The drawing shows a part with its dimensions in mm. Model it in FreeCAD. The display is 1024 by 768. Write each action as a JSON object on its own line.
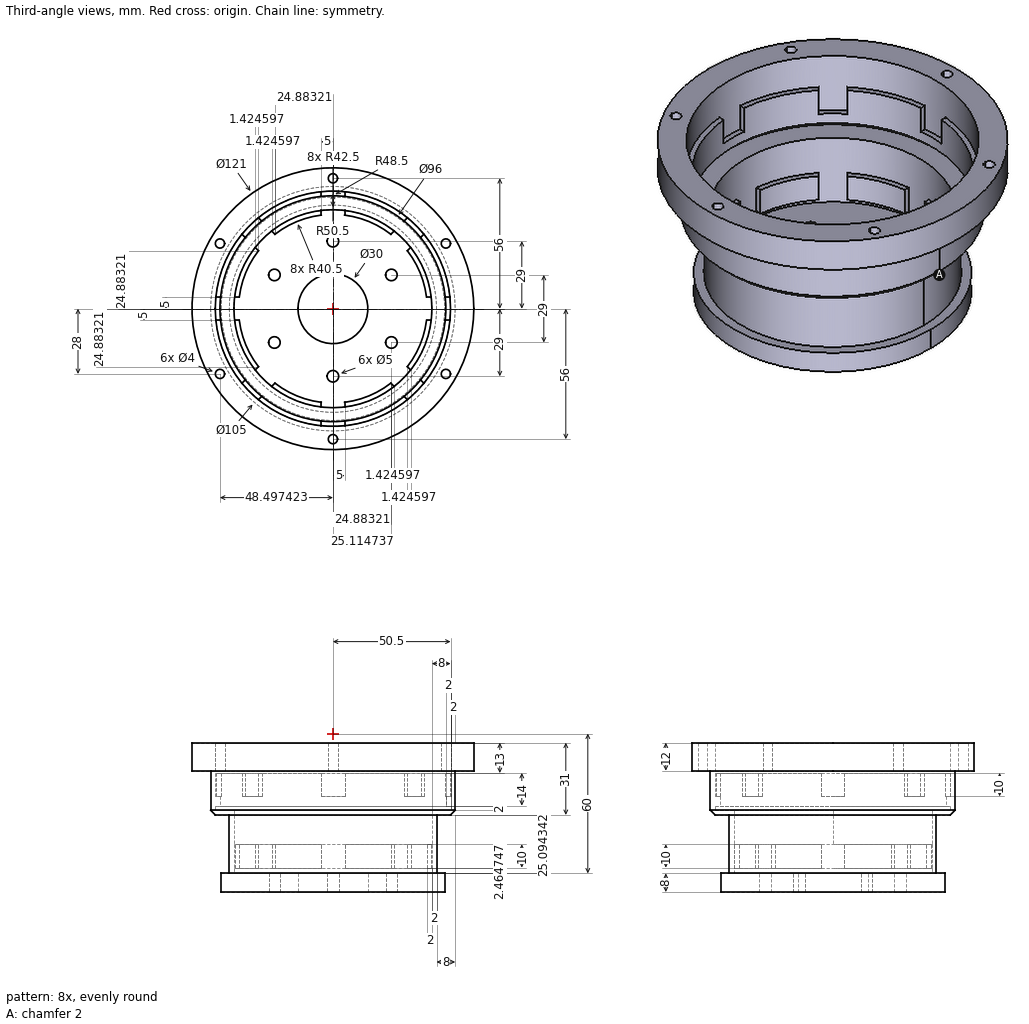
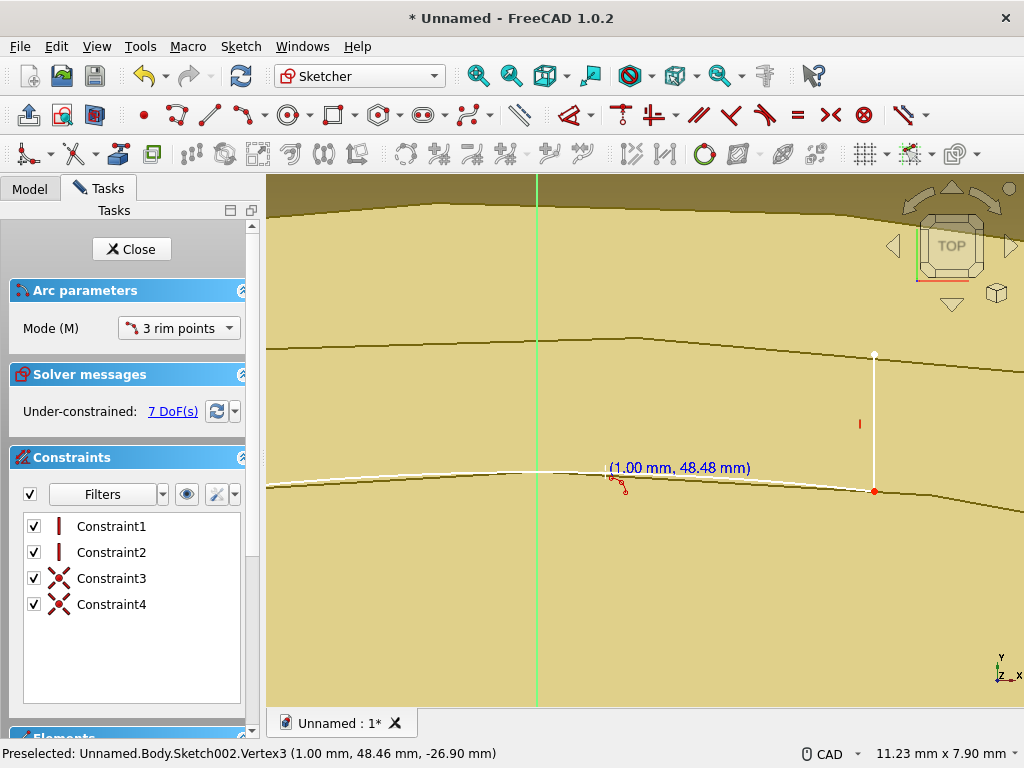
{"action": "scroll", "coordinate": [624, 474], "scroll_direction": "down", "scroll_amount": 3}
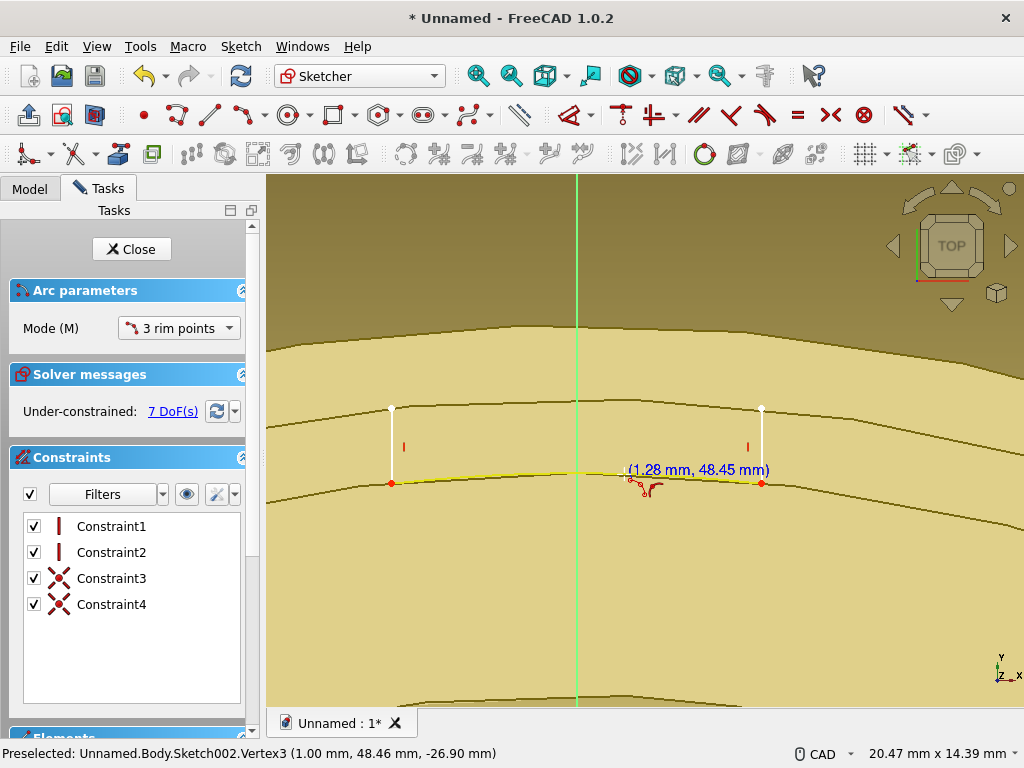
{"action": "left_click", "coordinate": [762, 409]}
{"action": "left_click", "coordinate": [392, 409]}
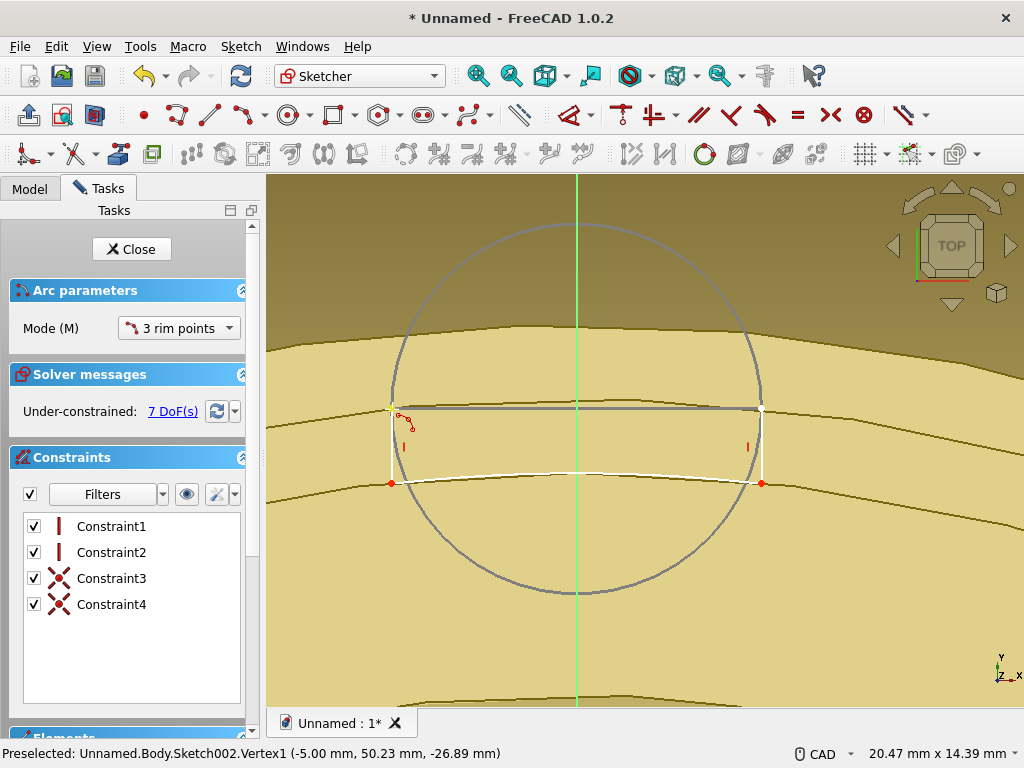
{"action": "scroll", "coordinate": [614, 399], "scroll_direction": "up", "scroll_amount": 3}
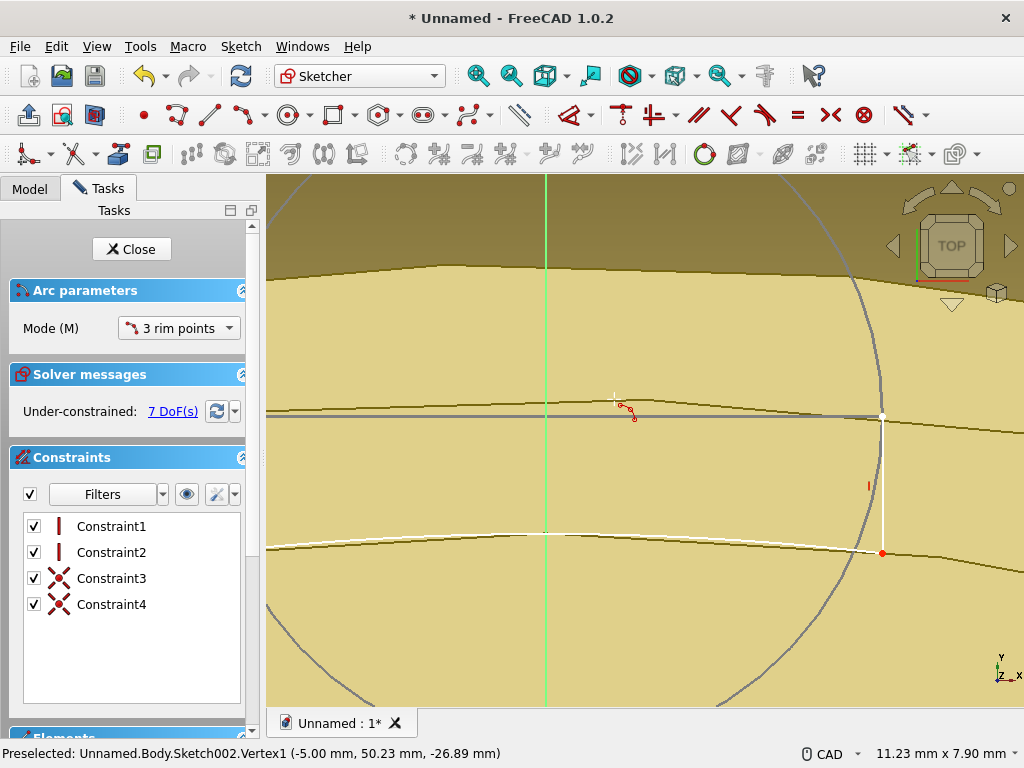
{"action": "left_click", "coordinate": [613, 399]}
{"action": "key", "text": "Escape"}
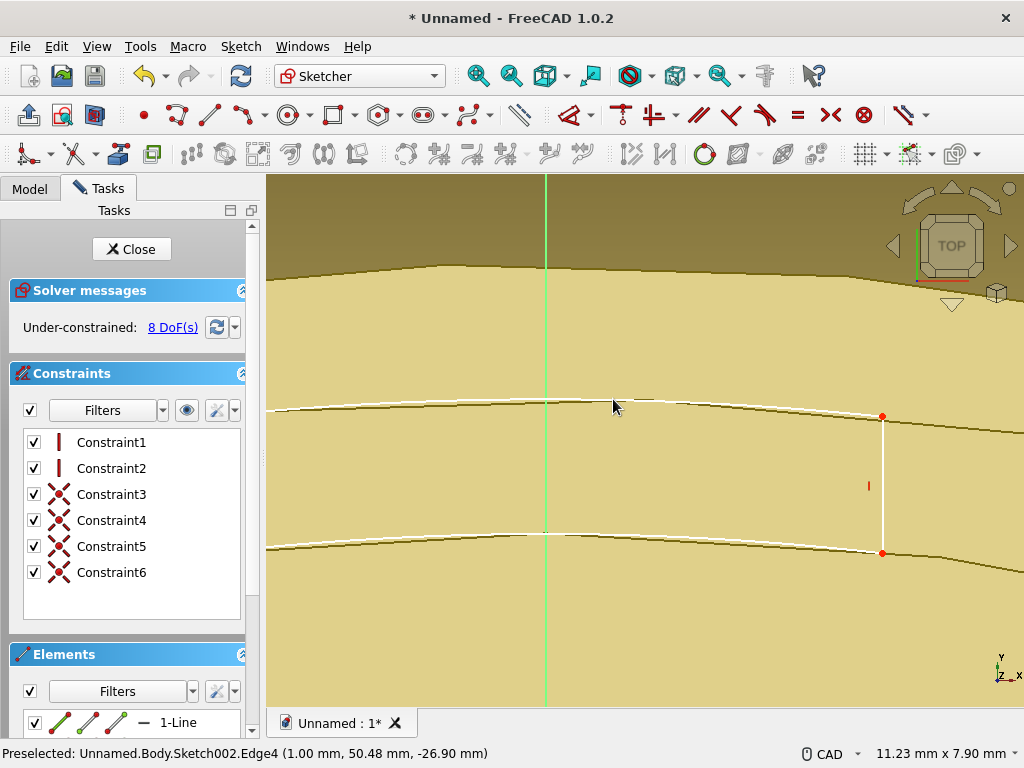
{"action": "left_click", "coordinate": [681, 537]}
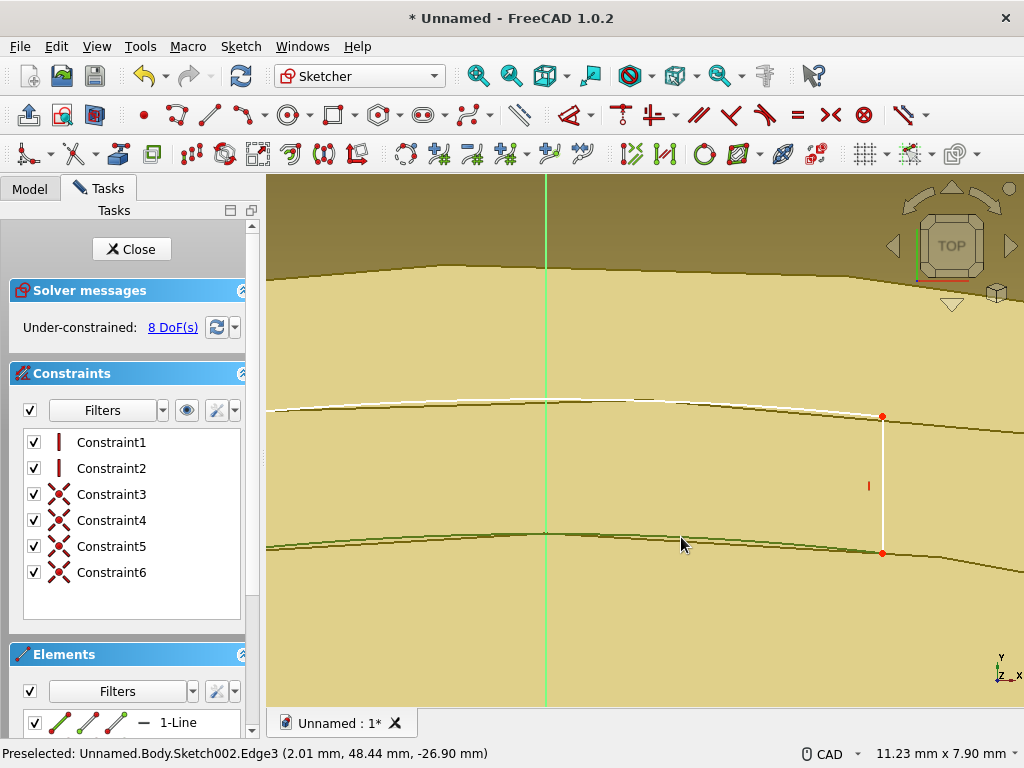
{"action": "left_click", "coordinate": [680, 402]}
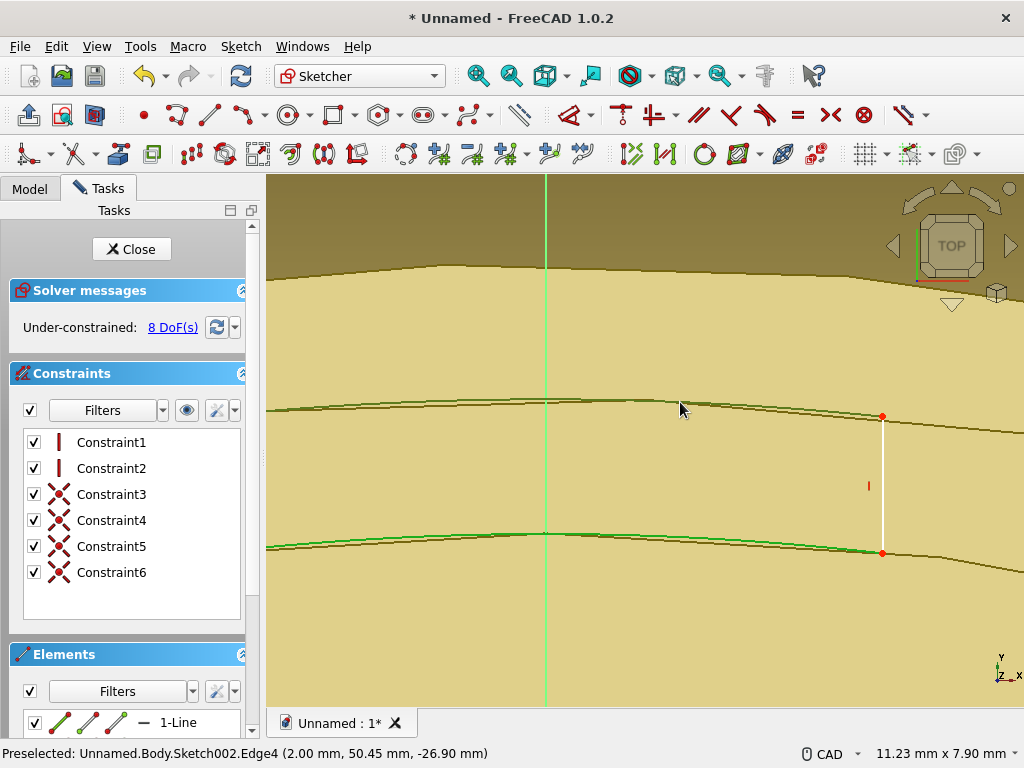
{"action": "key", "text": "c"}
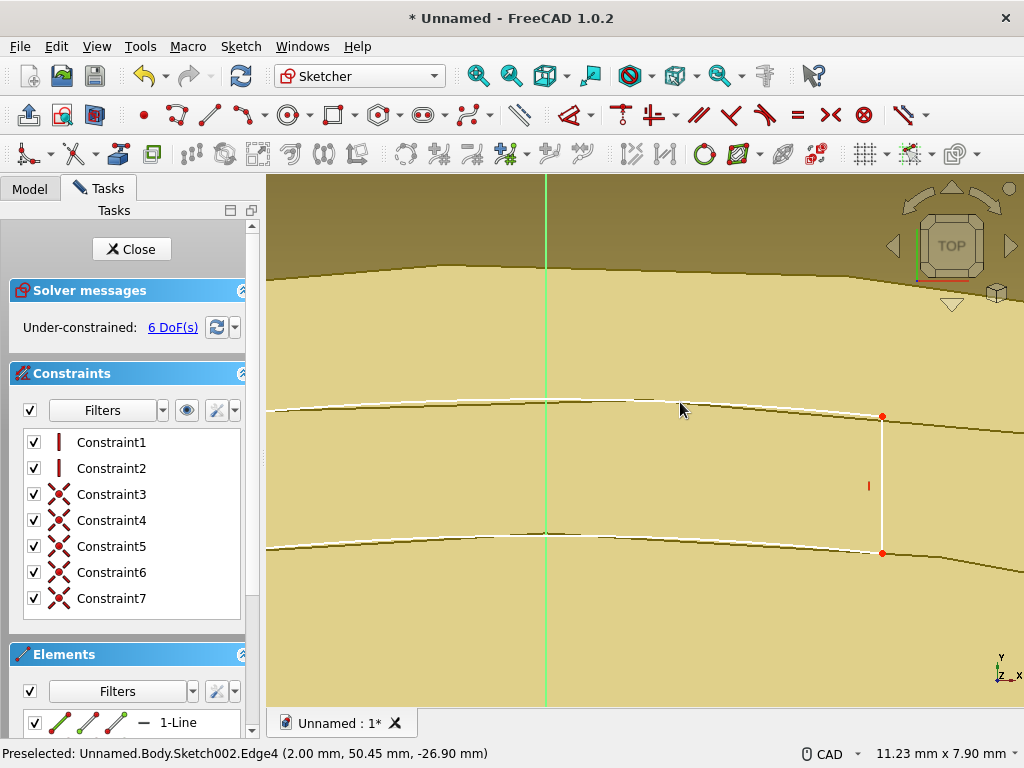
{"action": "scroll", "coordinate": [614, 399], "scroll_direction": "down", "scroll_amount": 3}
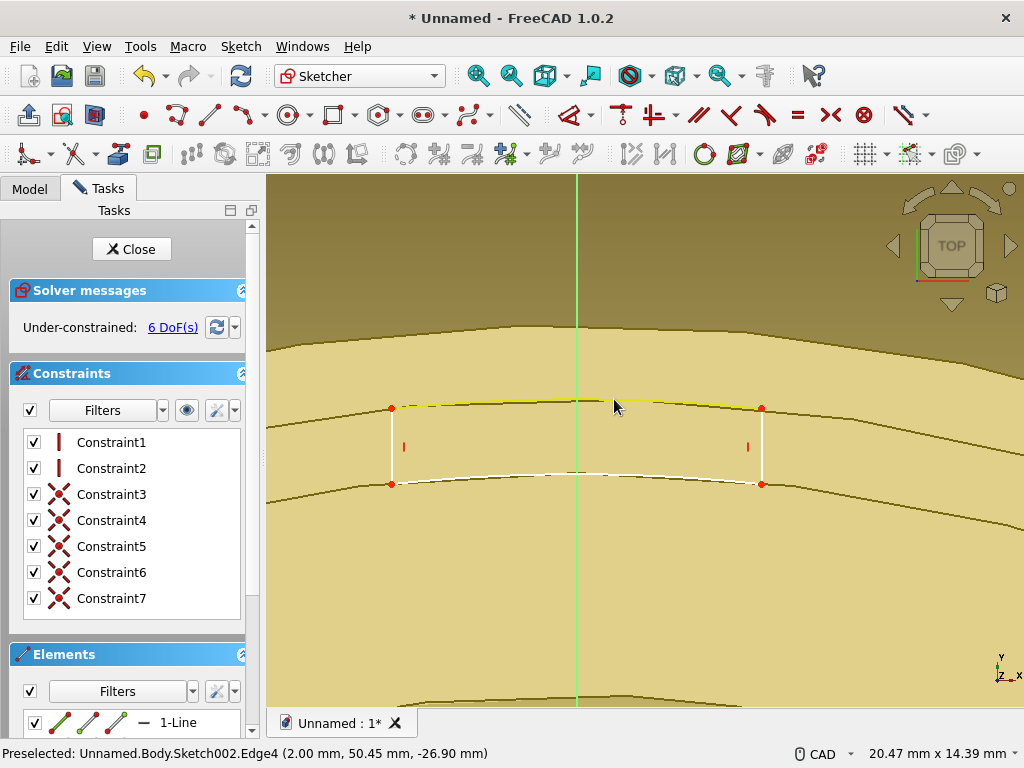
{"action": "scroll", "coordinate": [576, 219], "scroll_direction": "down", "scroll_amount": 8}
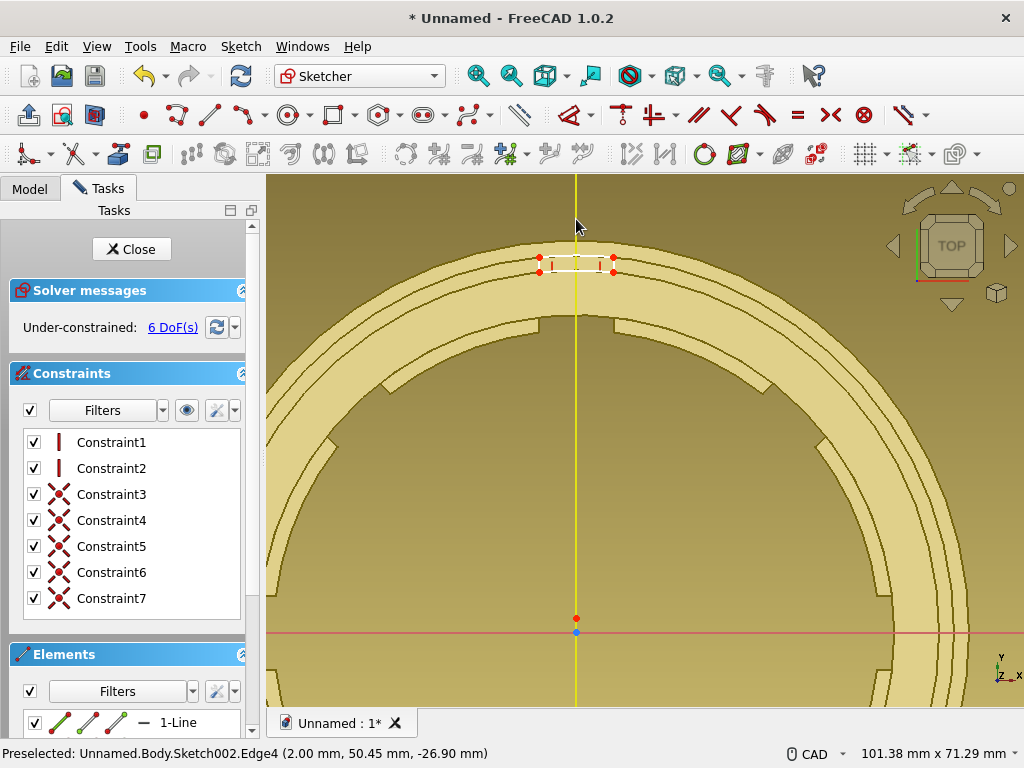
{"action": "left_click_drag", "start_coordinate": [566, 608], "coordinate": [586, 643]}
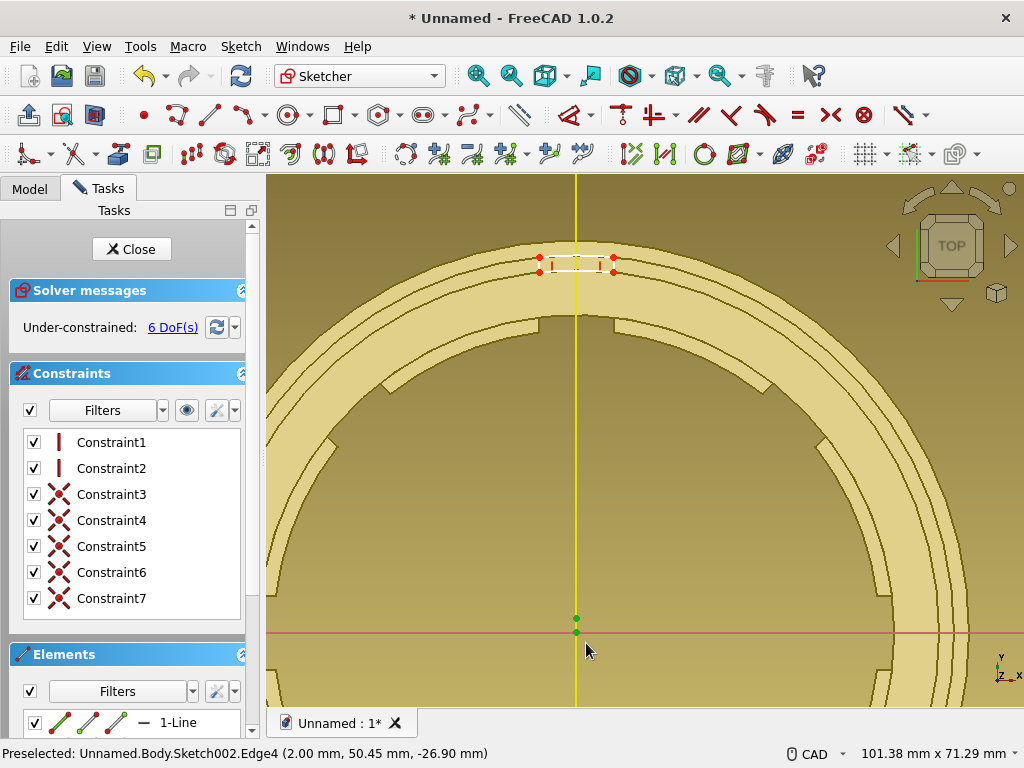
{"action": "key", "text": "c"}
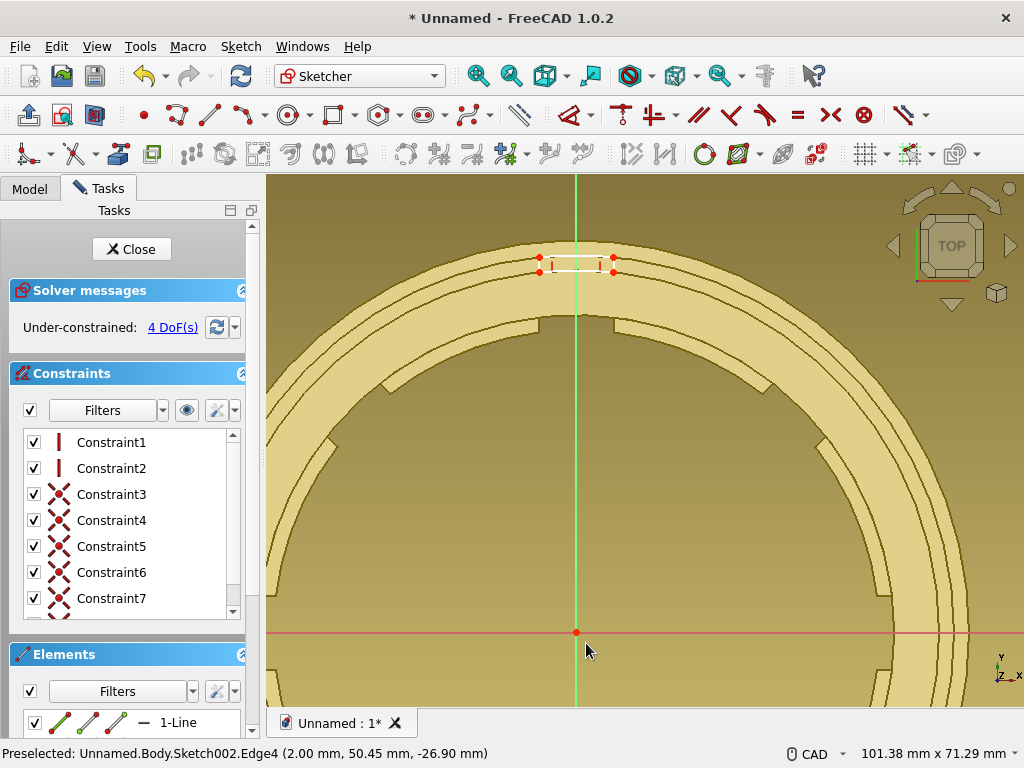
{"action": "key", "text": "d"}